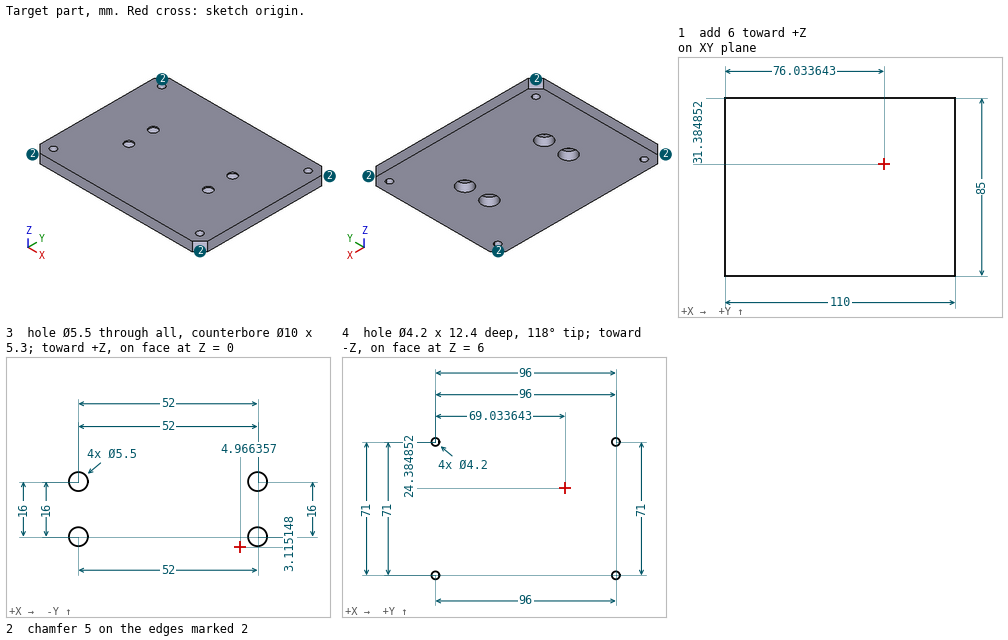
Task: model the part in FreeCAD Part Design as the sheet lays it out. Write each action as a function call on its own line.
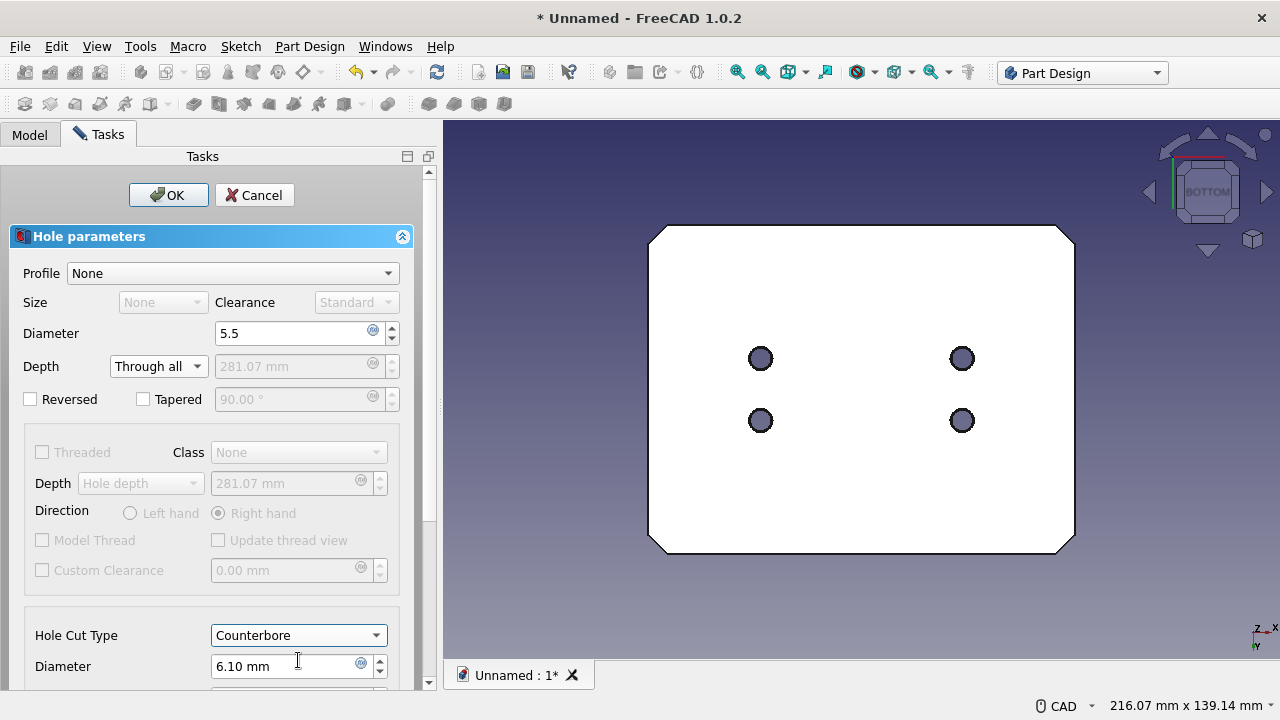
triple_click(292, 666)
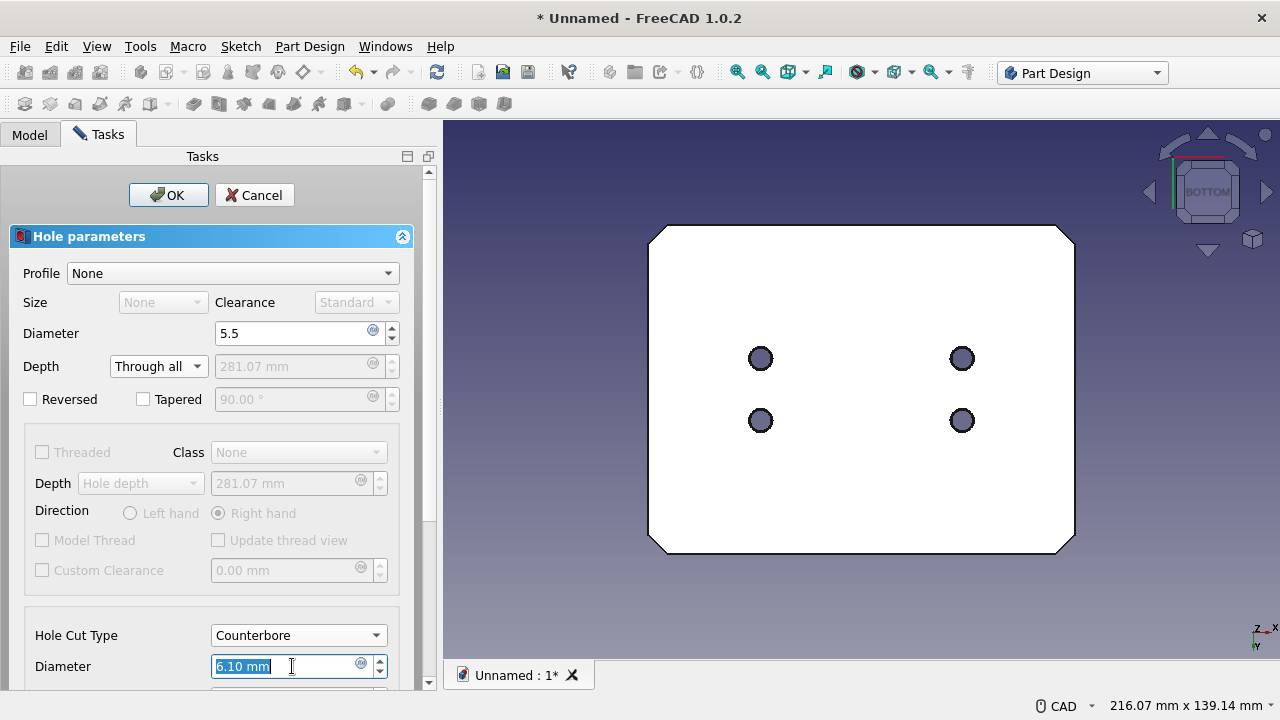
text(10)
key(Tab)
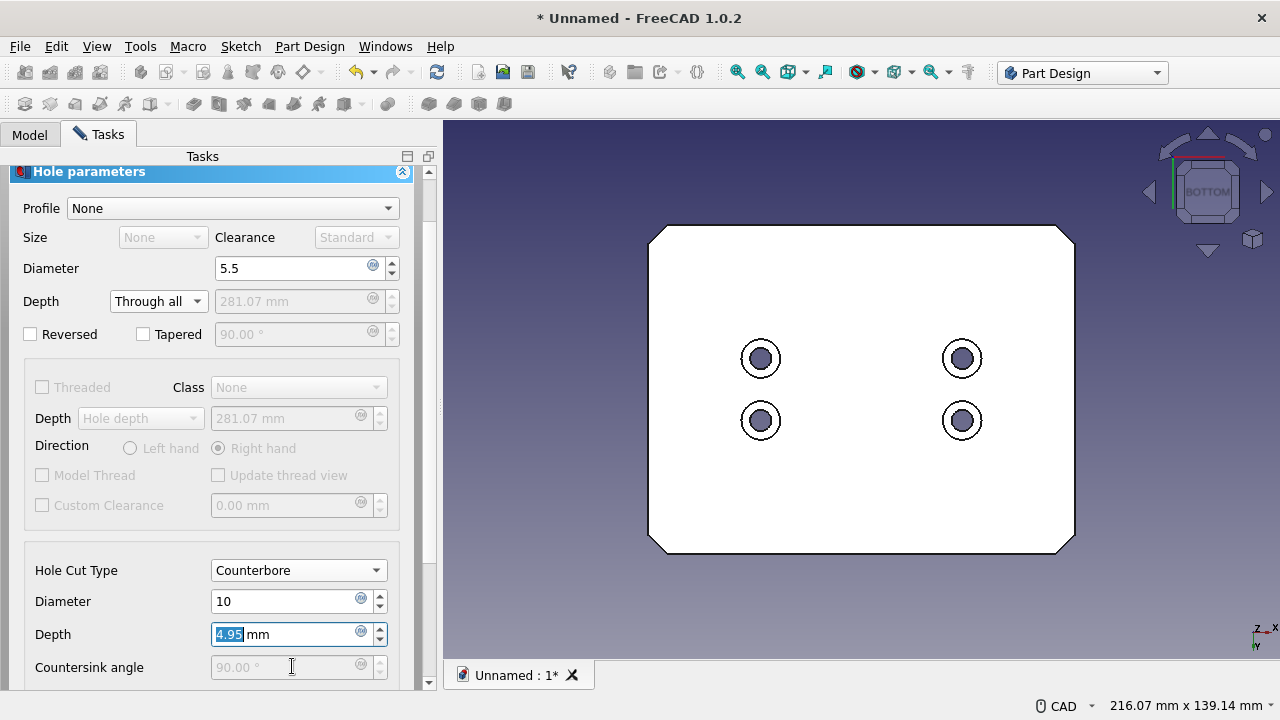
text(5.3)
key(Tab)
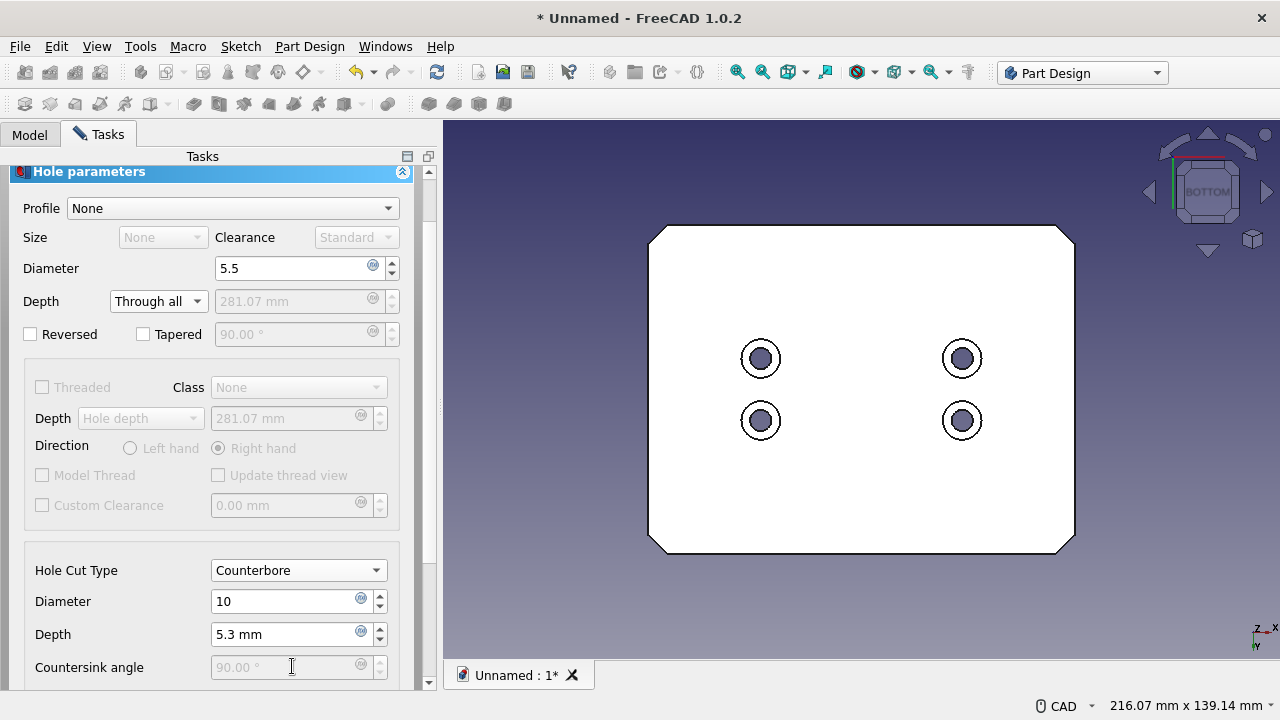
scroll(429, 428, up, 2)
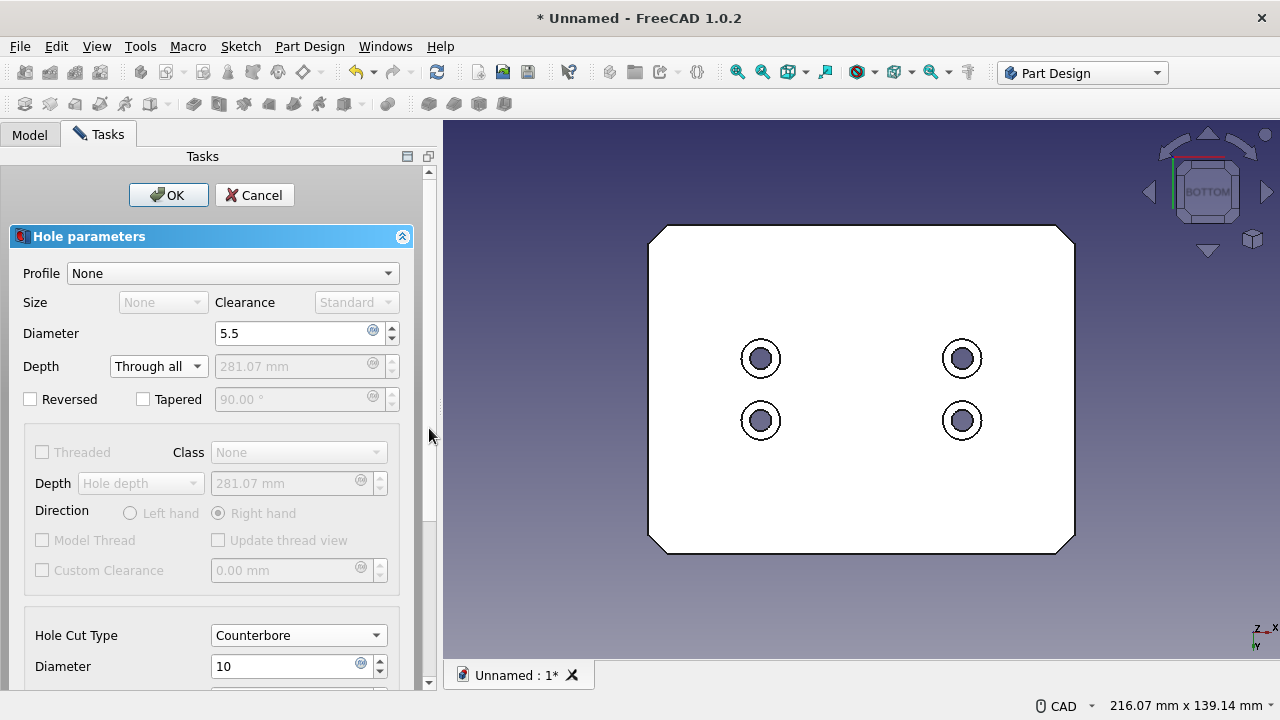
click(169, 195)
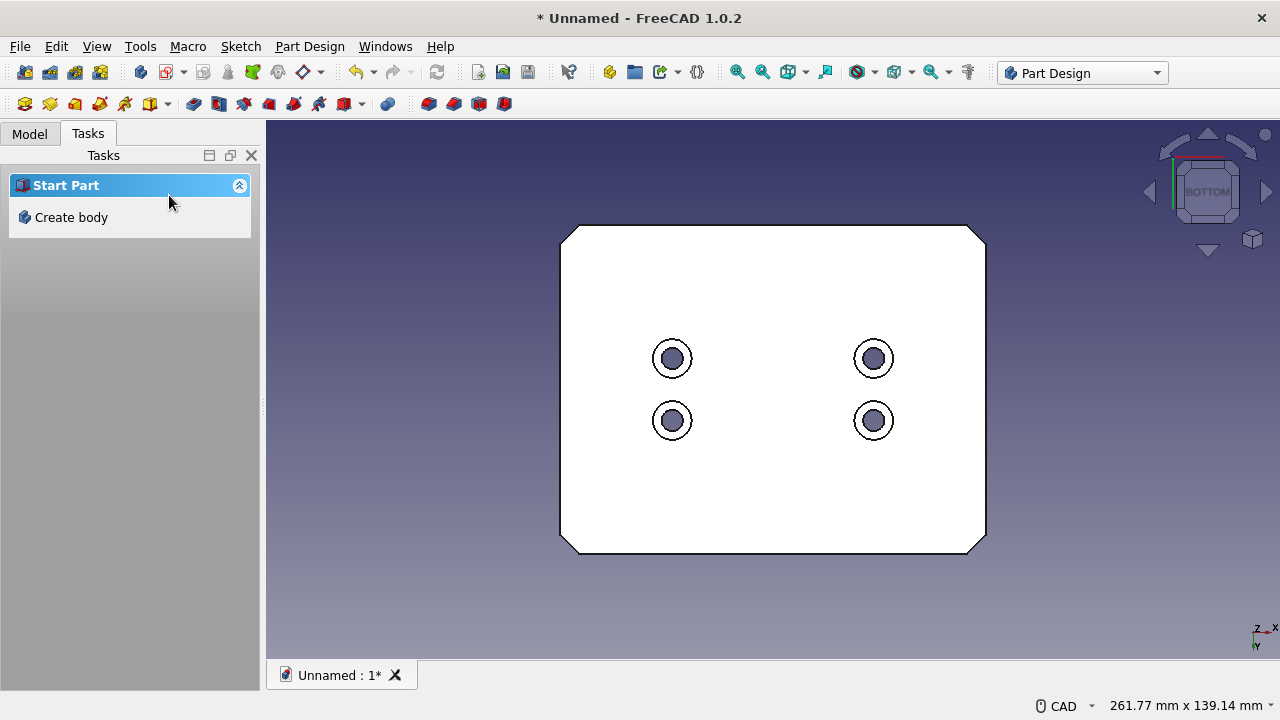
key(0)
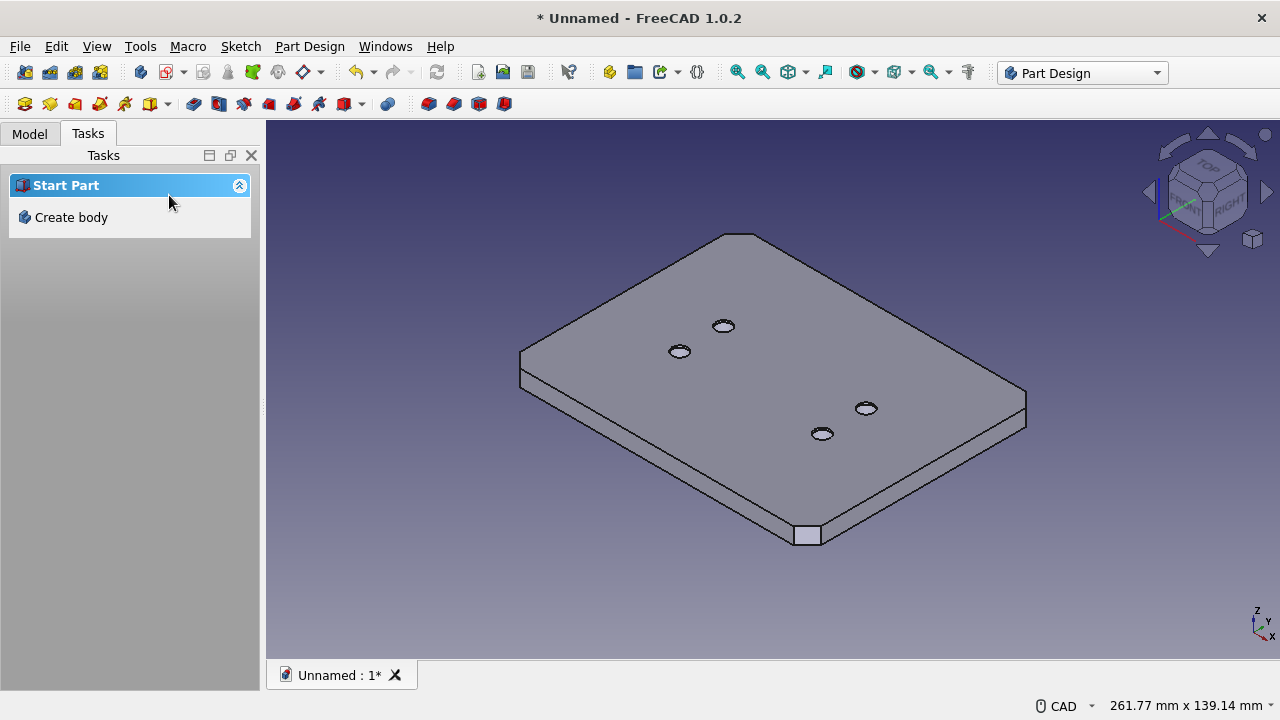
click(773, 379)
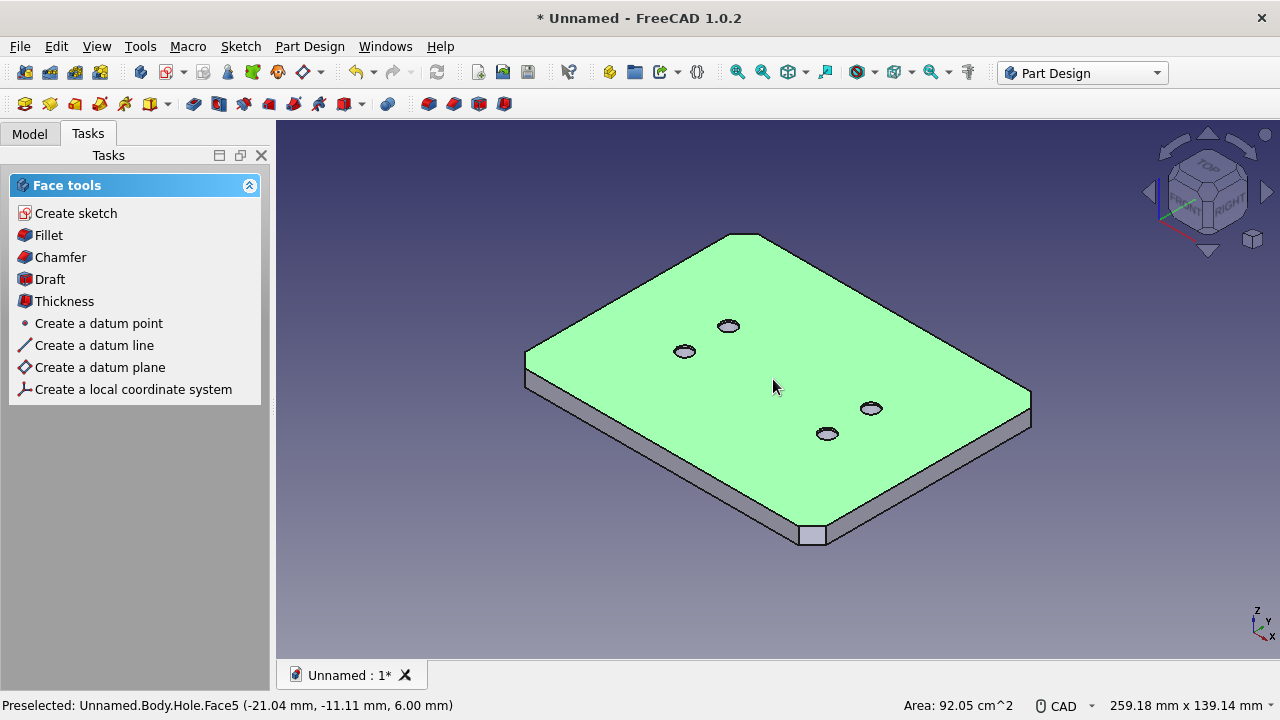
click(166, 72)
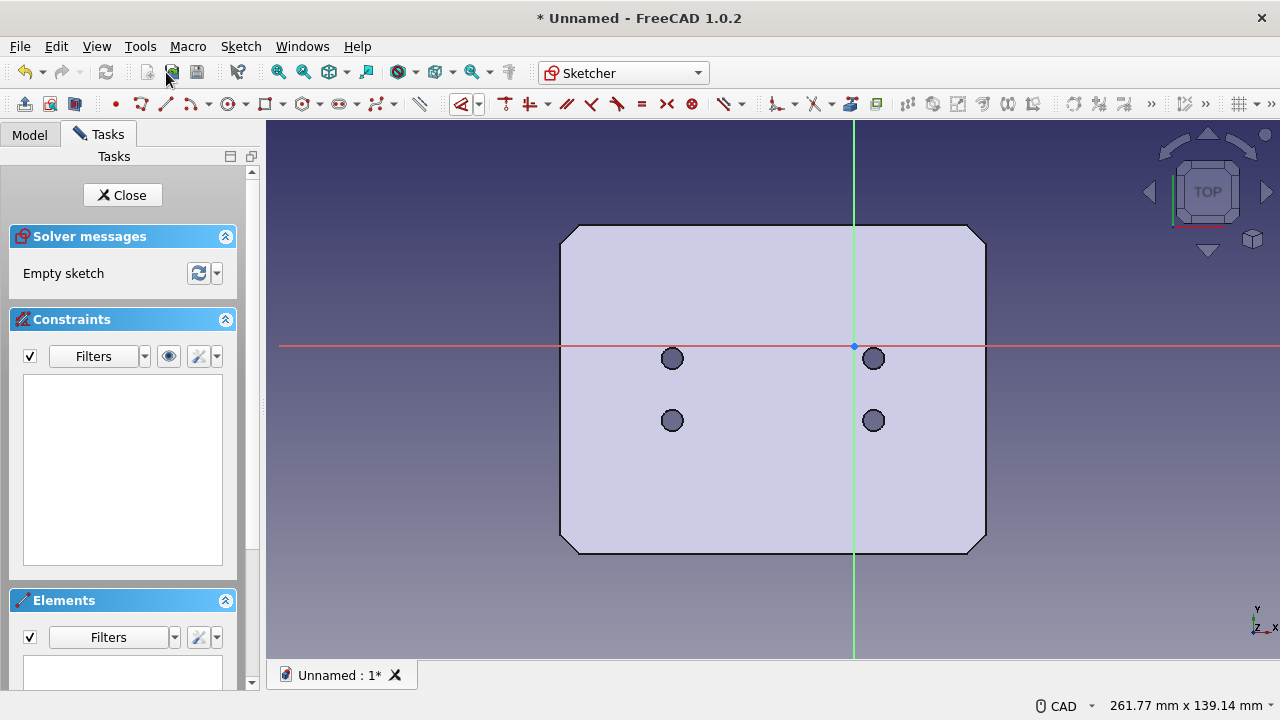
key(g)
key(c)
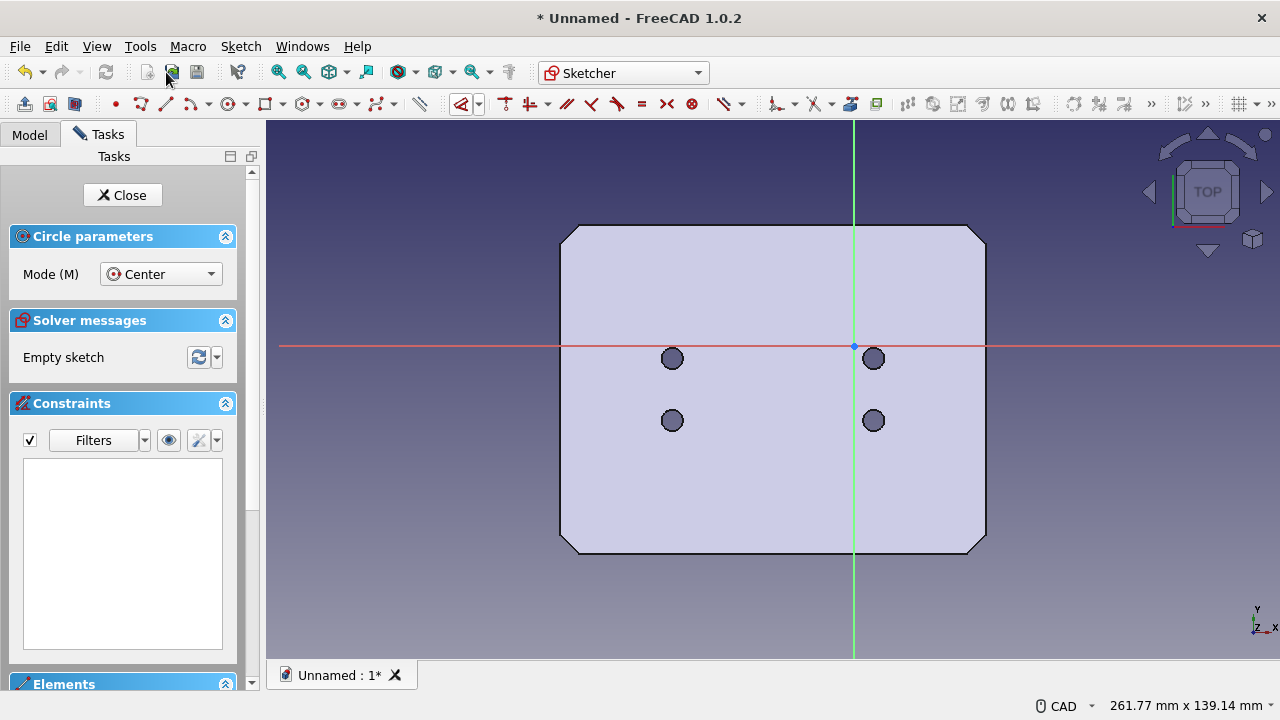
scroll(587, 252, up, 6)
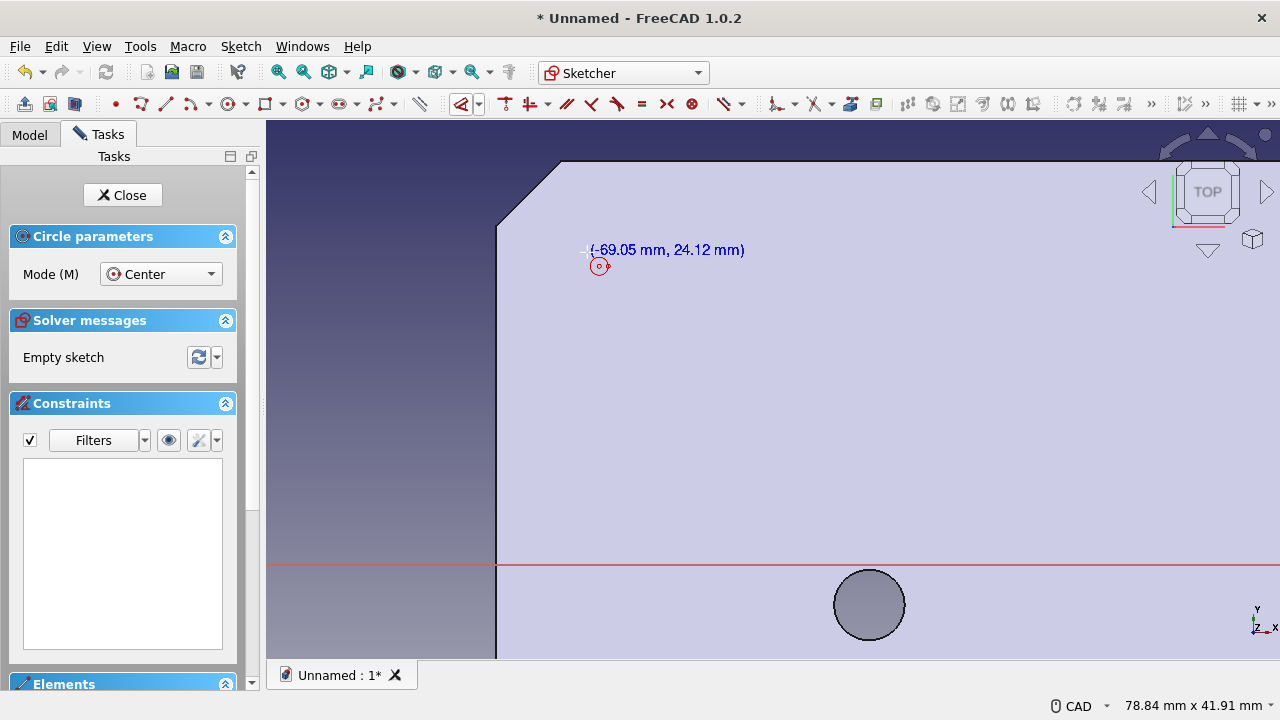
click(586, 251)
move(606, 232)